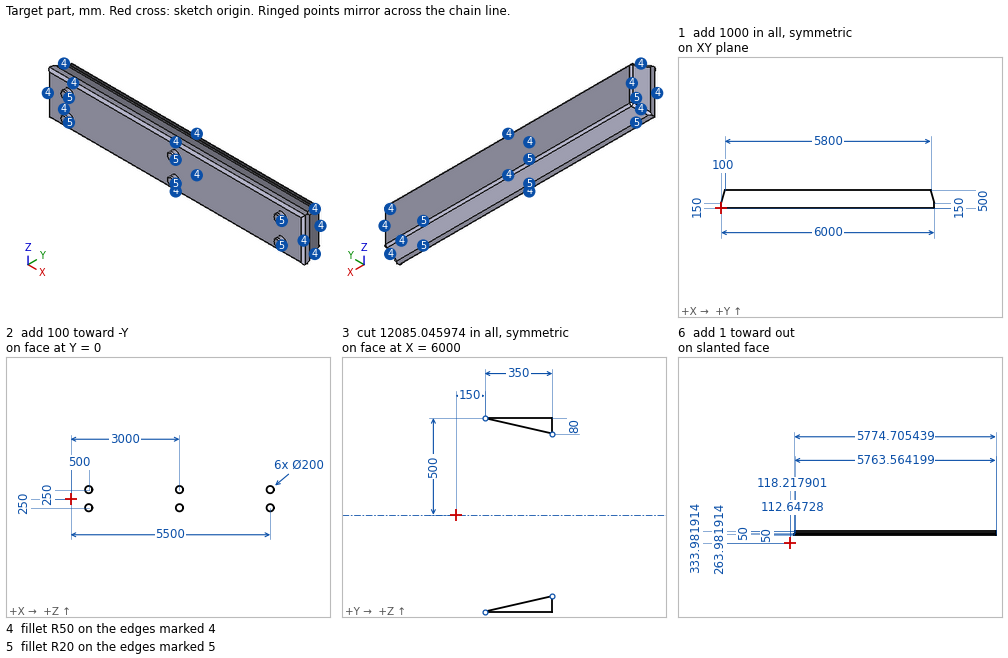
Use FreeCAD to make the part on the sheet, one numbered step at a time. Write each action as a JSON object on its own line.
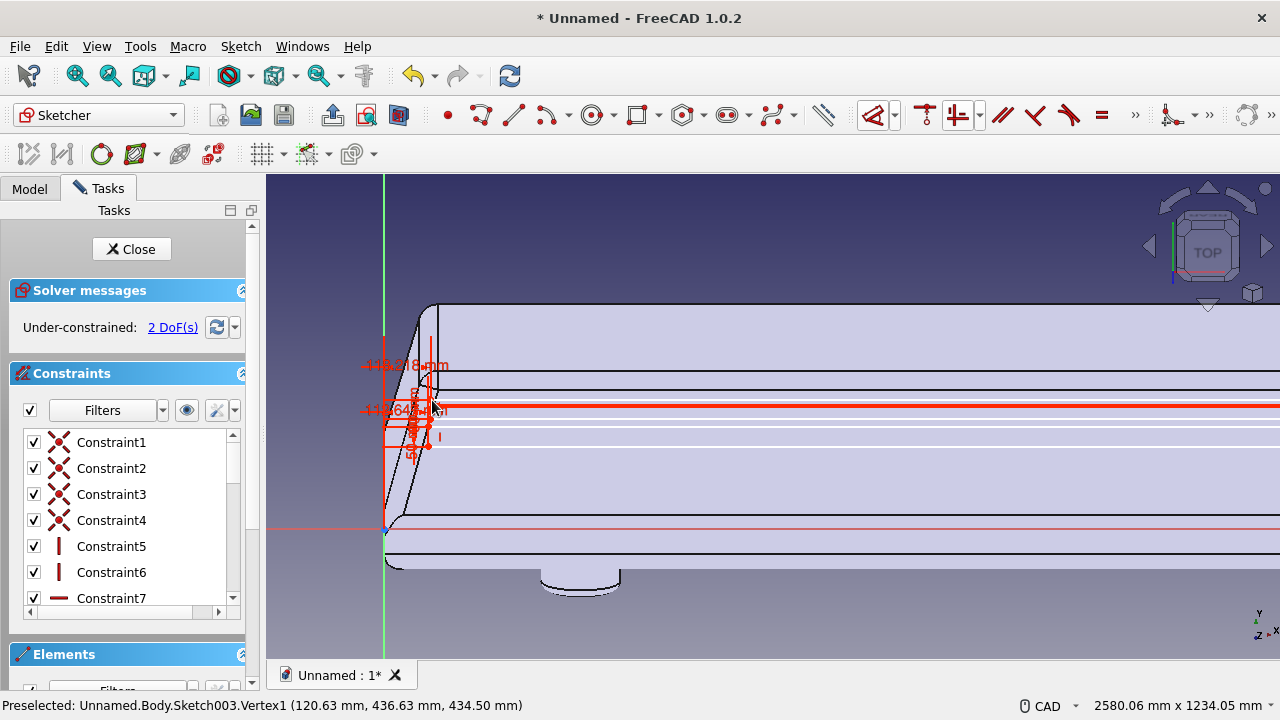
{"action": "left_click", "coordinate": [431, 400]}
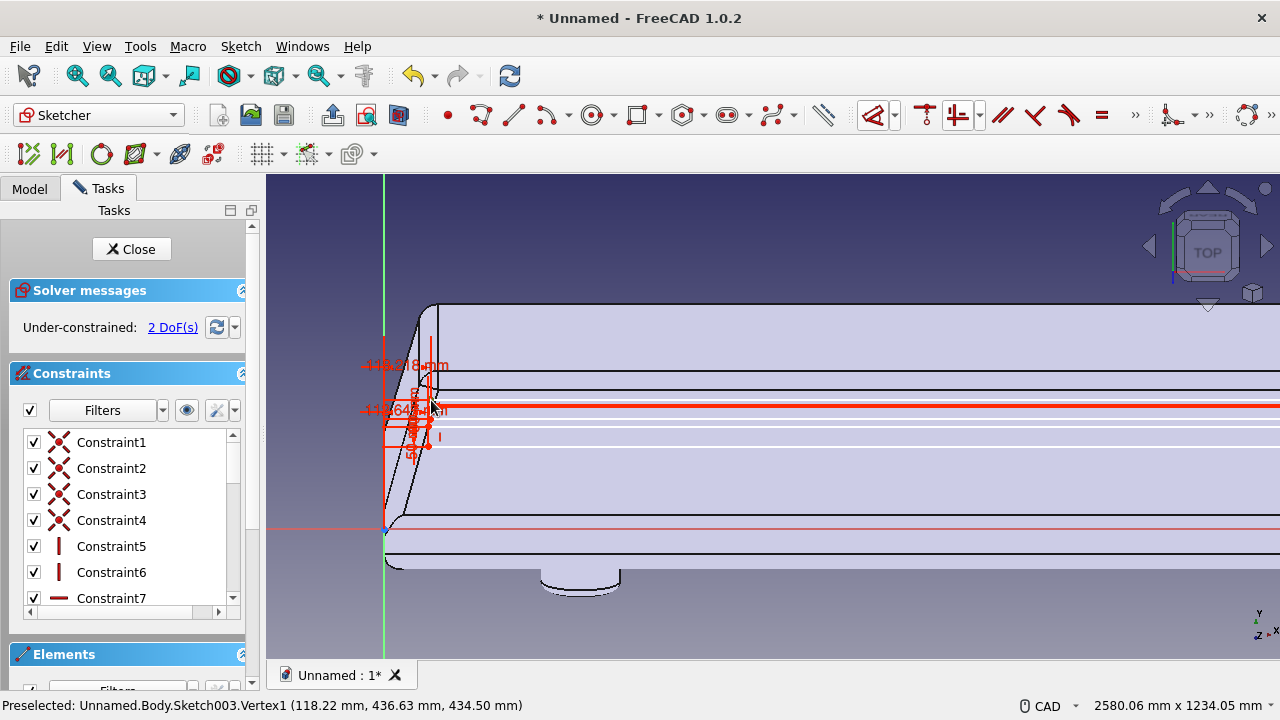
{"action": "left_click", "coordinate": [894, 116]}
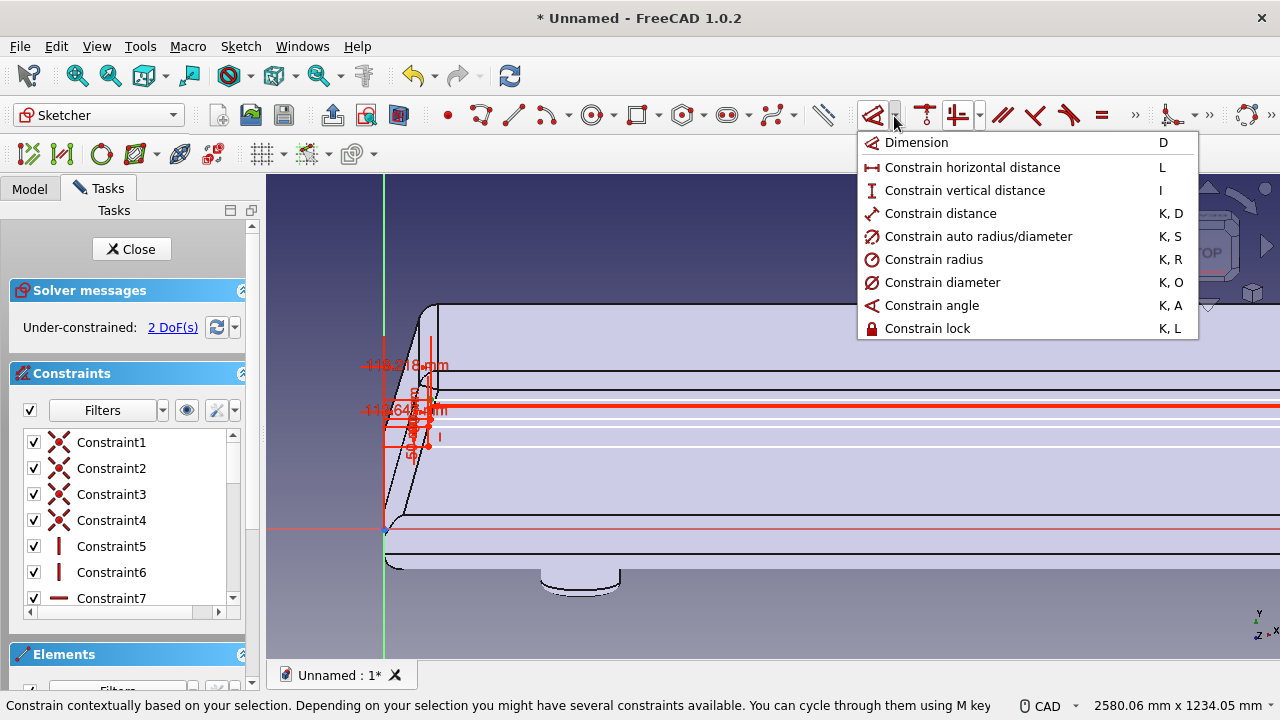
{"action": "left_click", "coordinate": [1028, 190]}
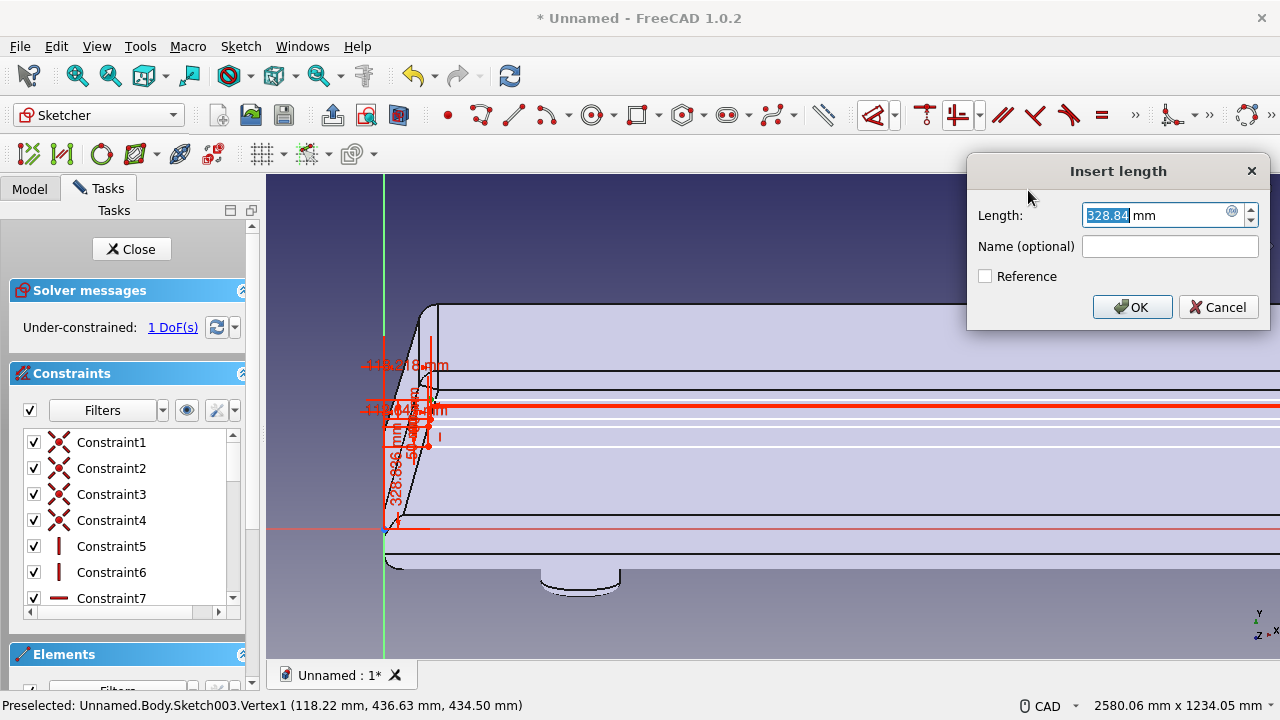
{"action": "type", "text": "333.981914"}
{"action": "key", "text": "Return"}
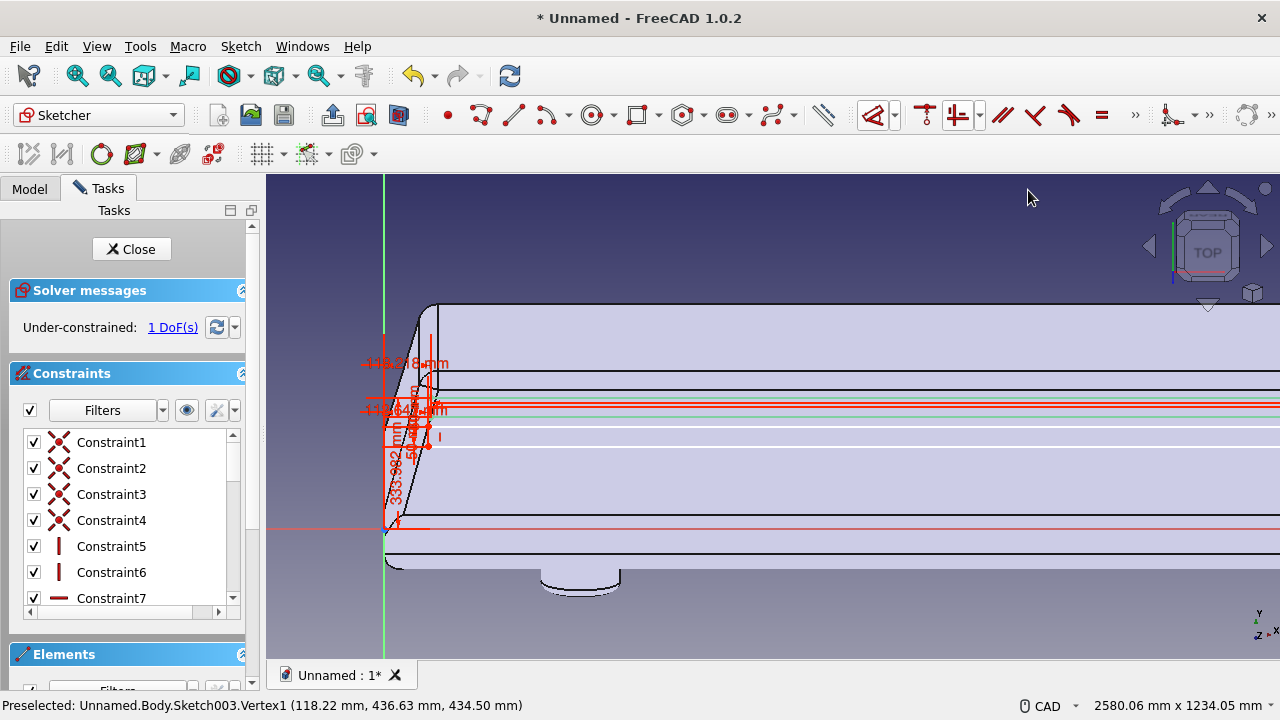
{"action": "scroll", "coordinate": [428, 427], "scroll_direction": "up", "scroll_amount": 2}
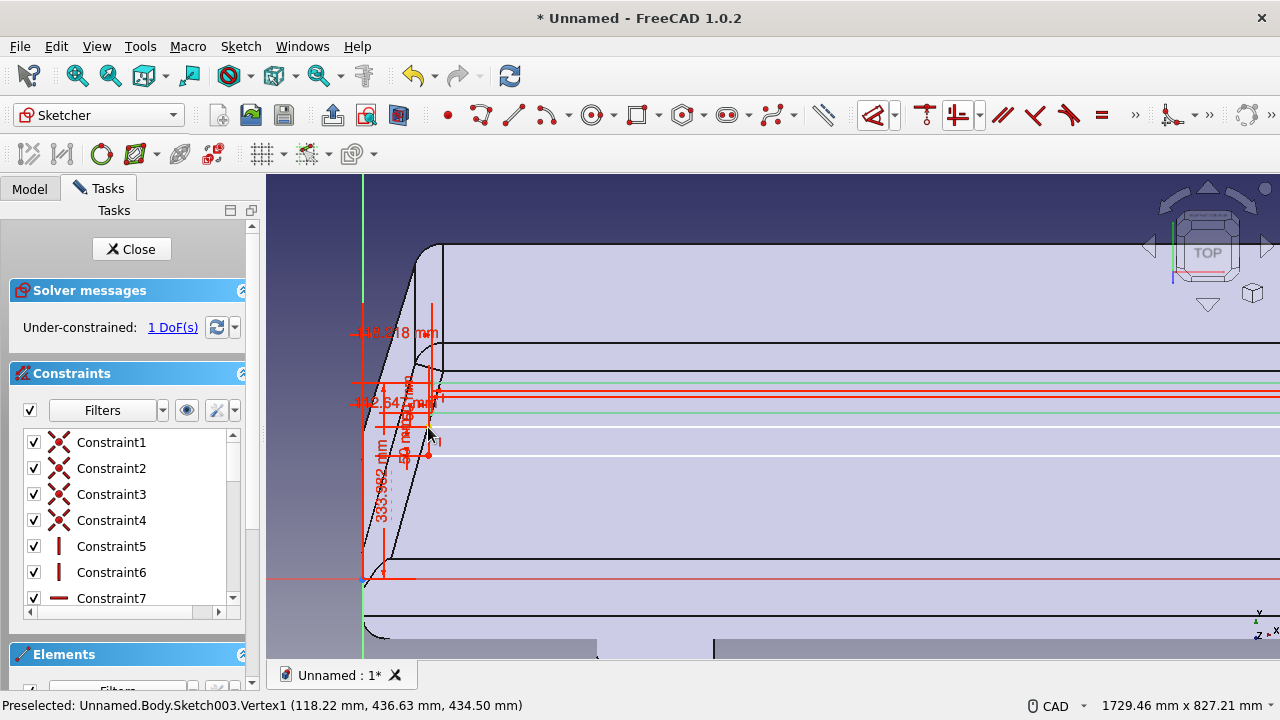
{"action": "left_click", "coordinate": [429, 427]}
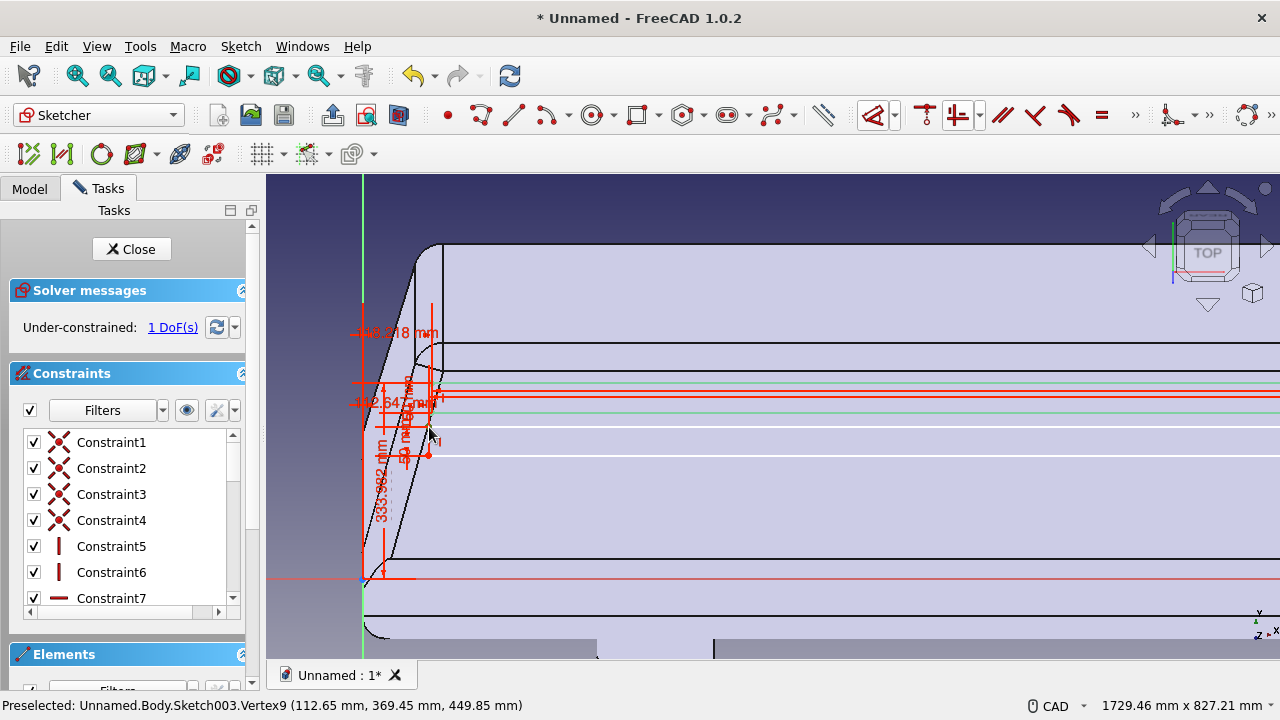
{"action": "left_click", "coordinate": [894, 116]}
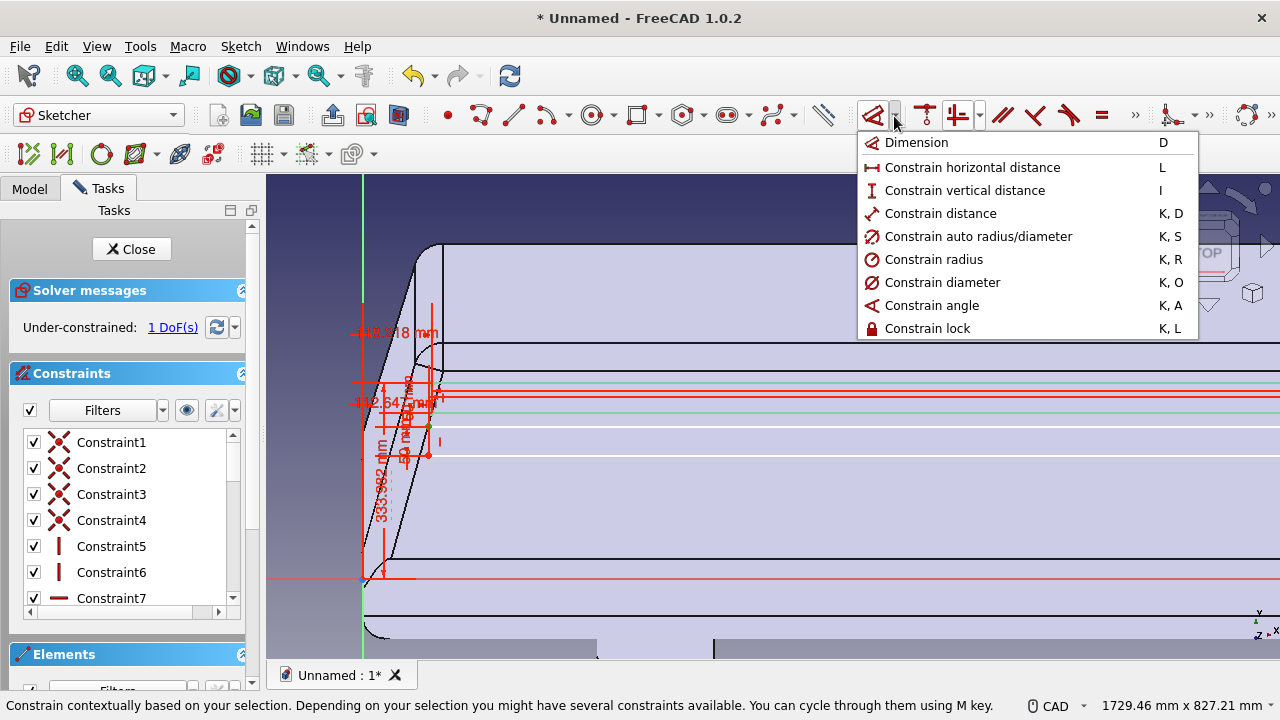
{"action": "left_click", "coordinate": [1028, 190]}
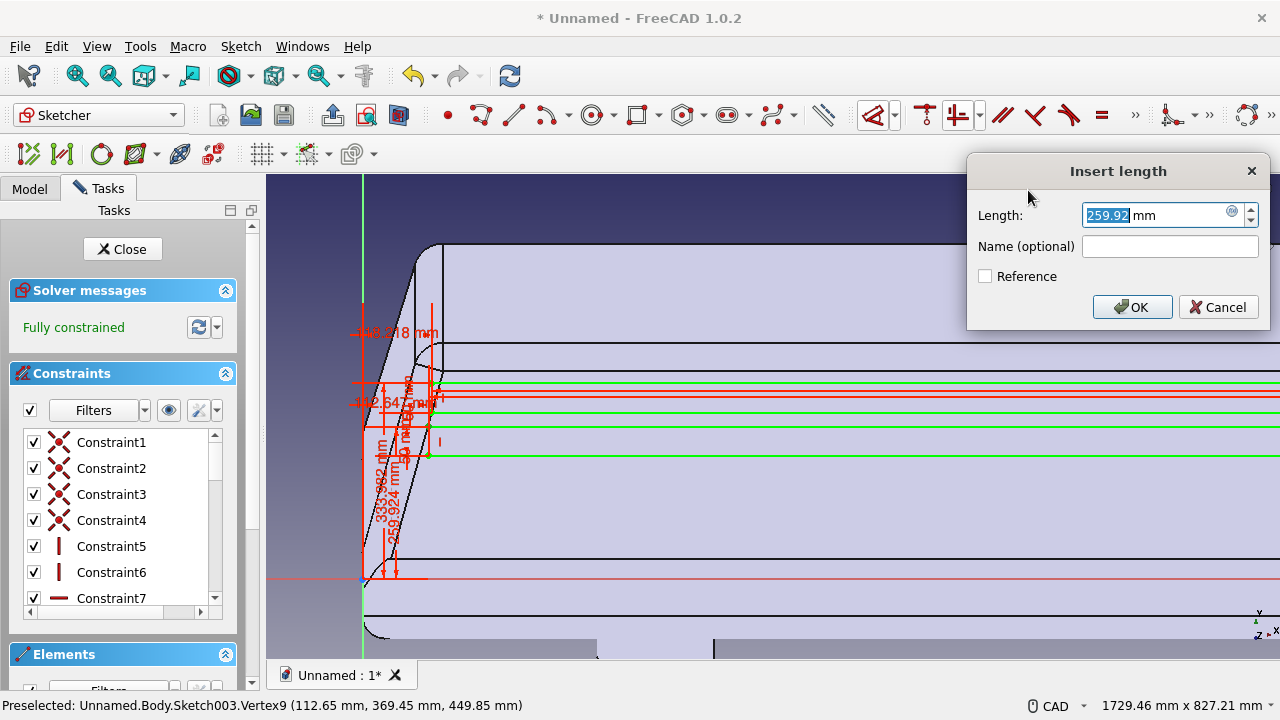
{"action": "type", "text": "263.981914"}
{"action": "key", "text": "Return"}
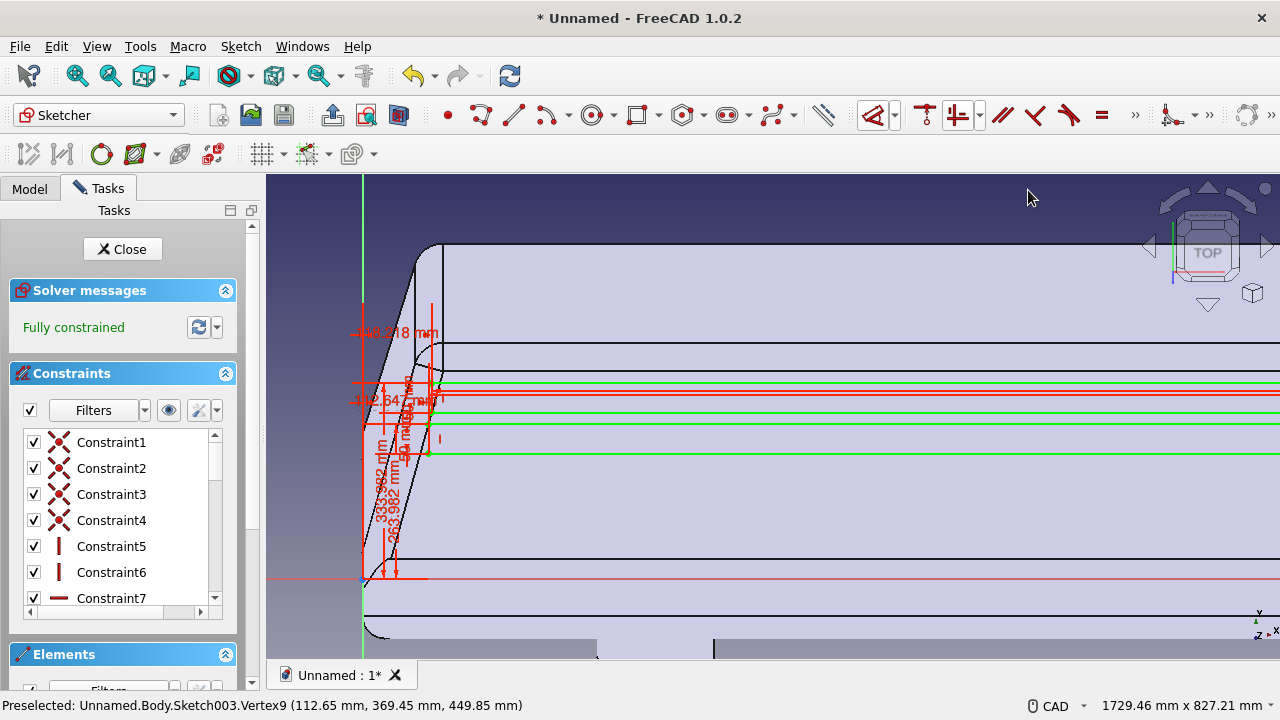
{"action": "left_click", "coordinate": [123, 249]}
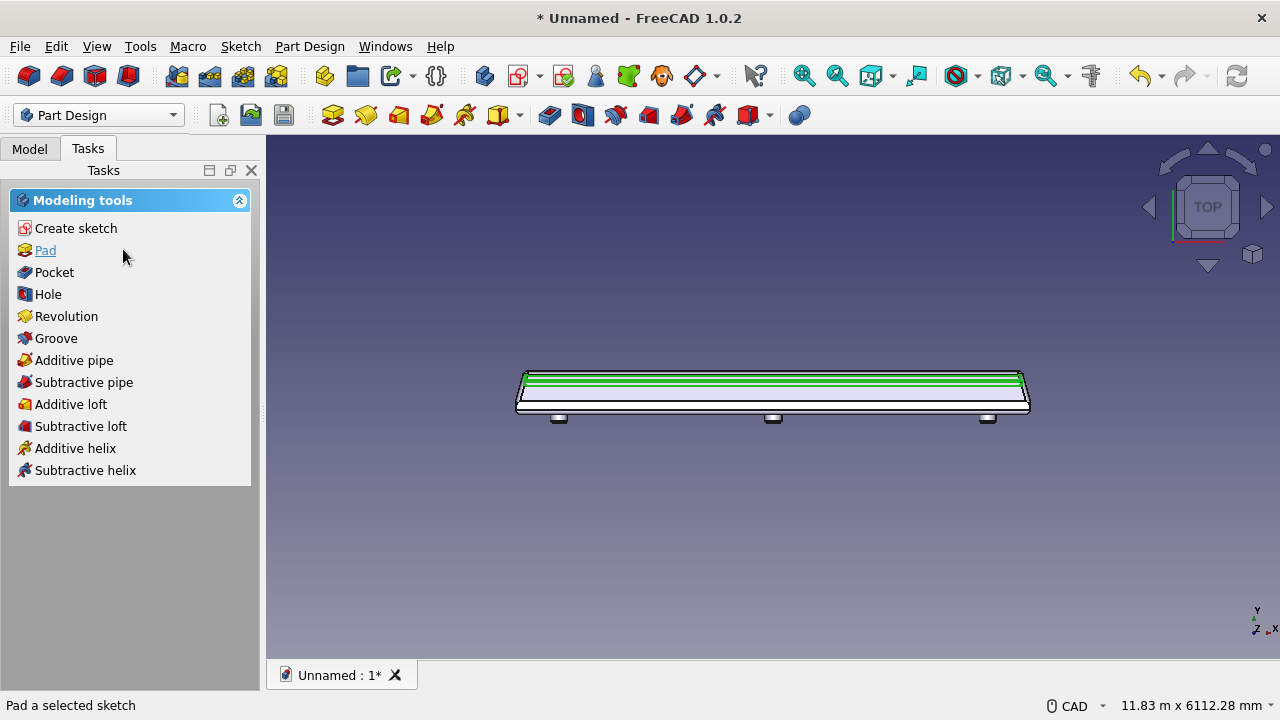
{"action": "left_click", "coordinate": [333, 116]}